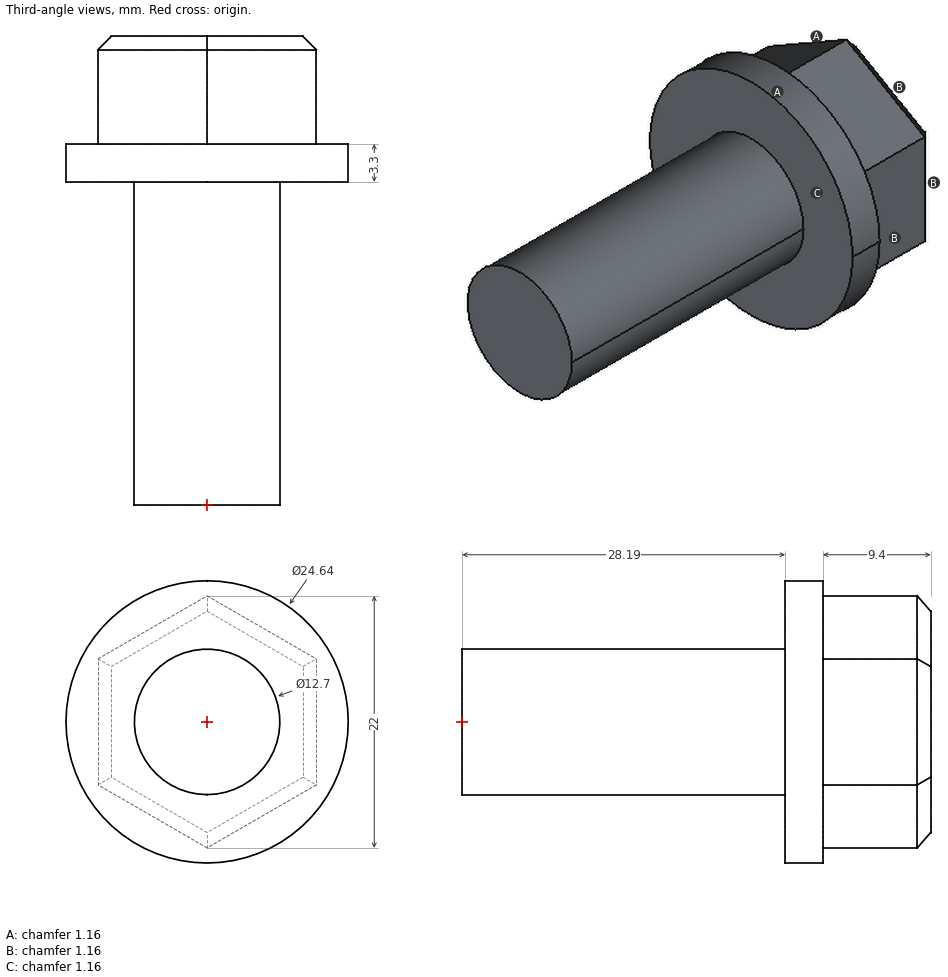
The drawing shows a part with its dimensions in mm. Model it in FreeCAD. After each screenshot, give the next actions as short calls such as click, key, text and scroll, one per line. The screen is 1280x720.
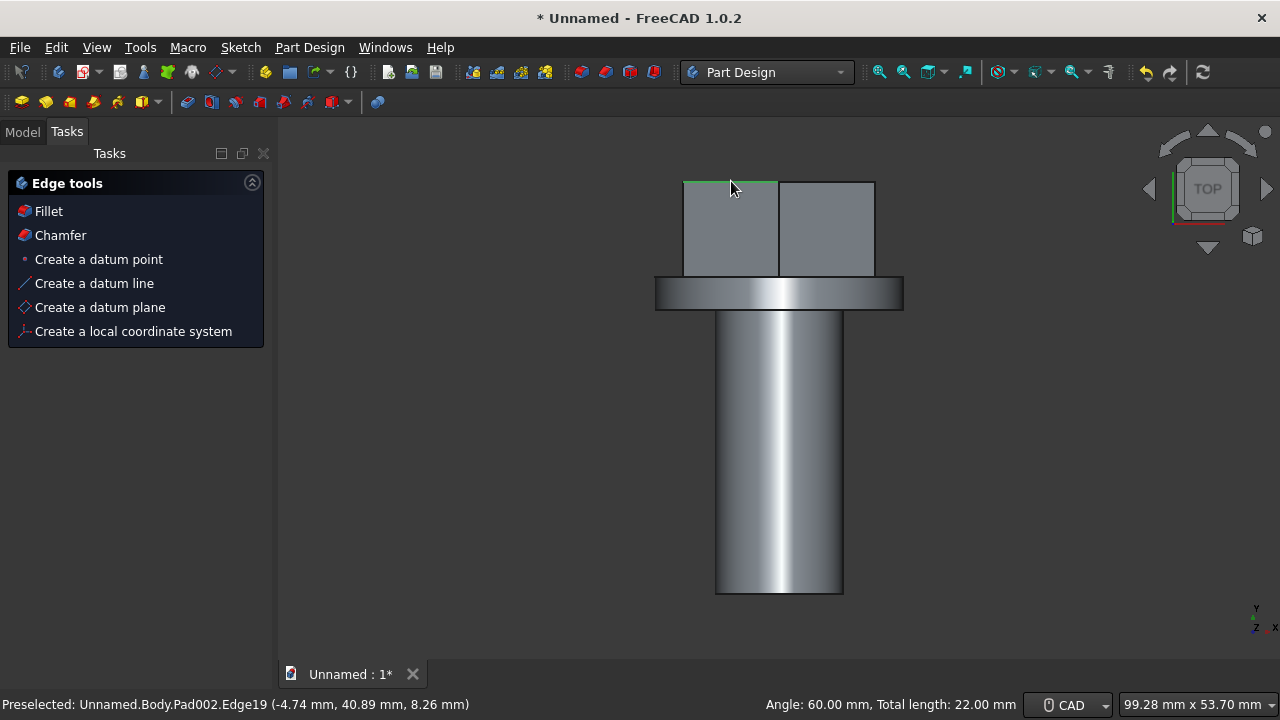
click(606, 72)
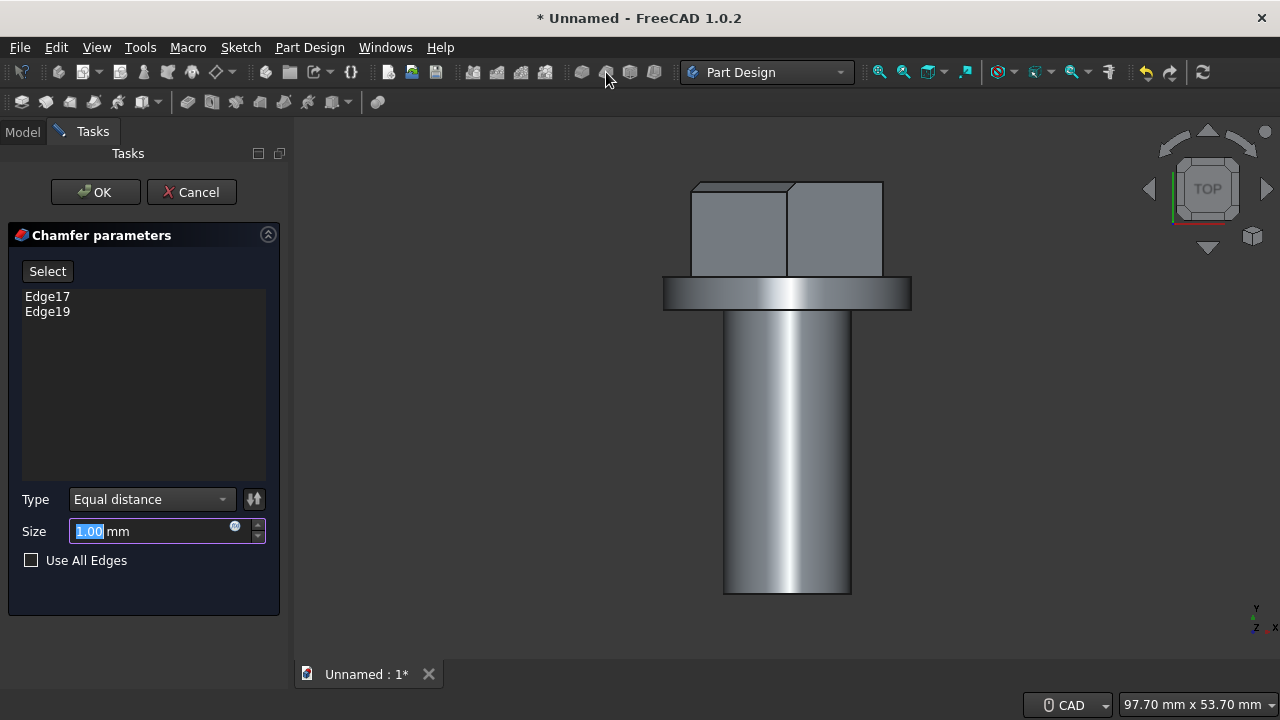
text(1.16)
key(Tab)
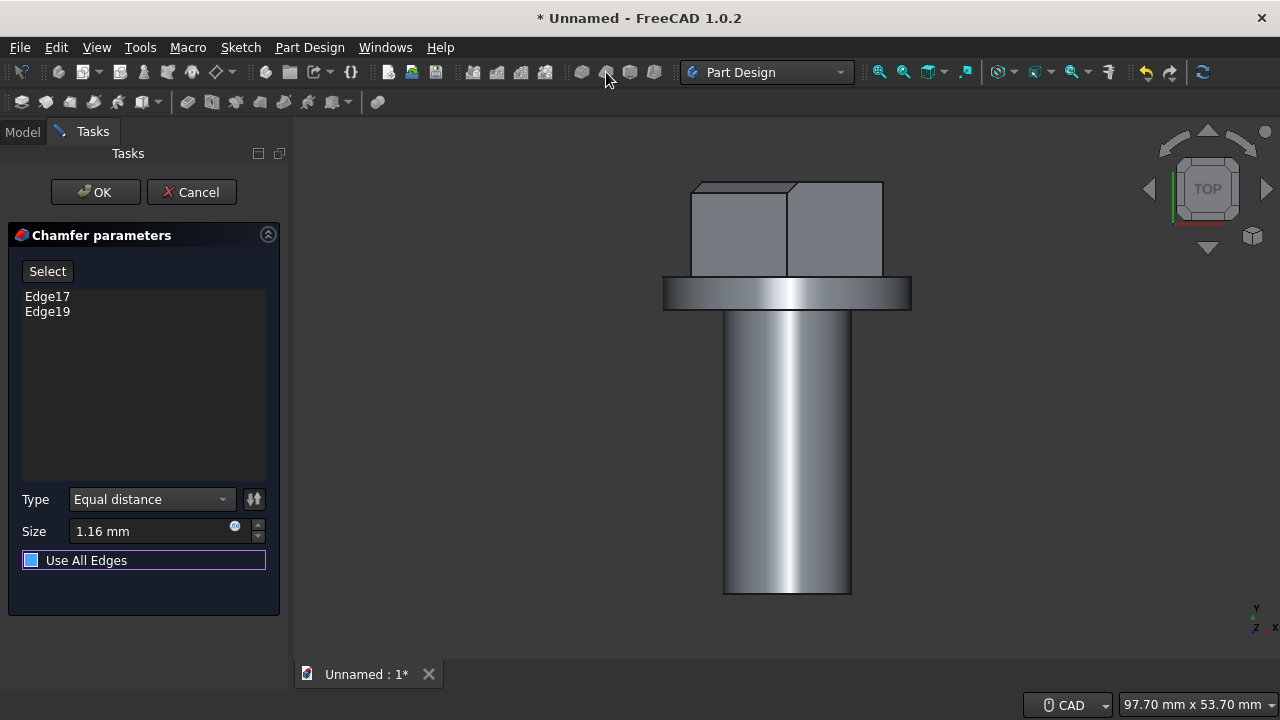
click(96, 192)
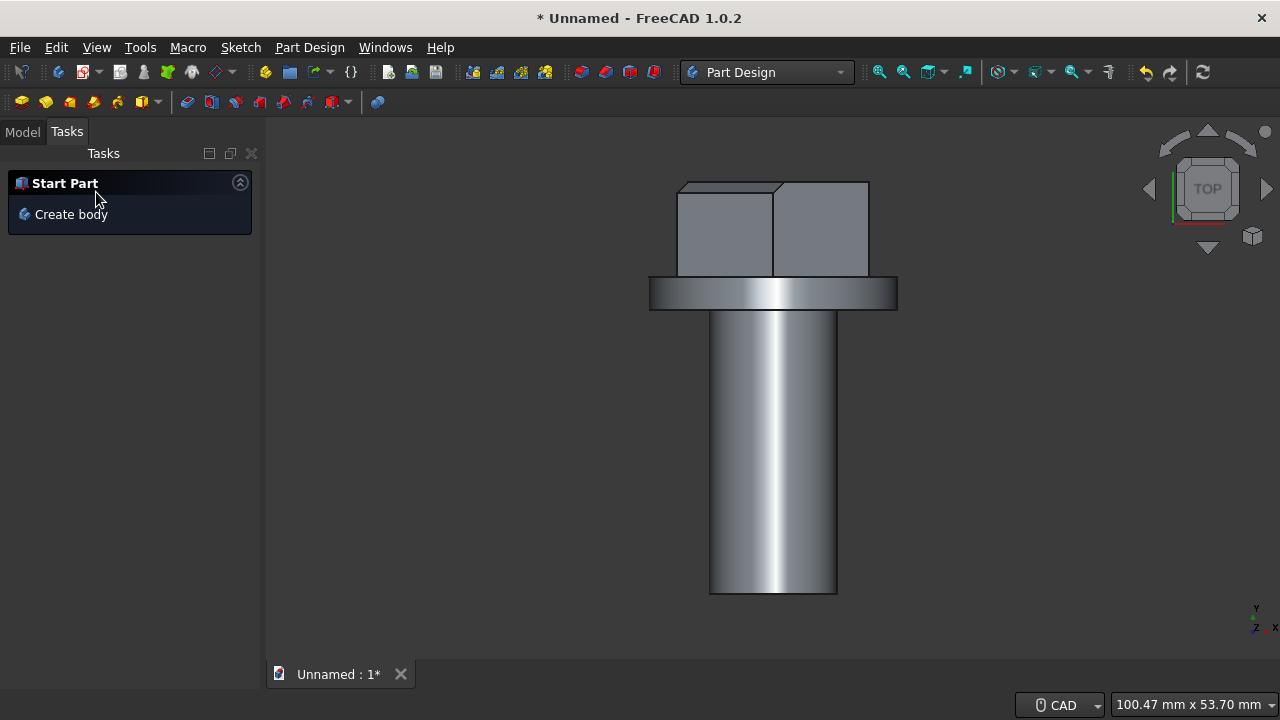
click(827, 181)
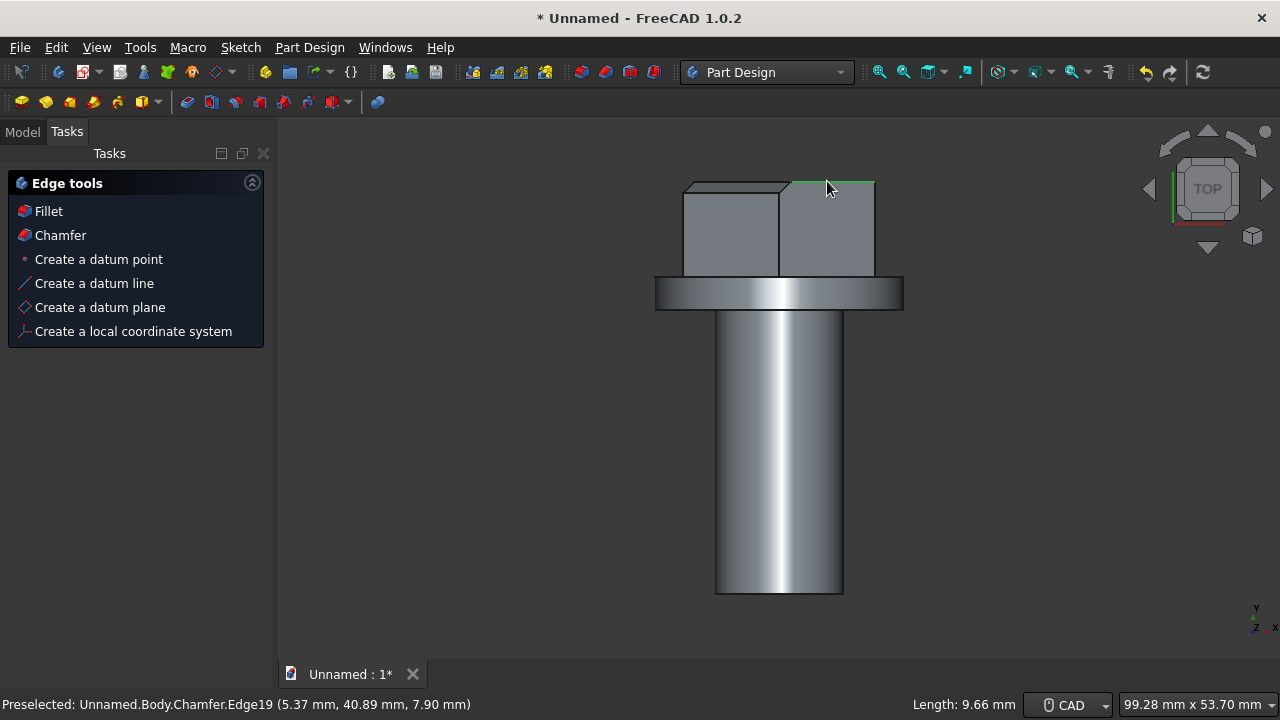
key(0)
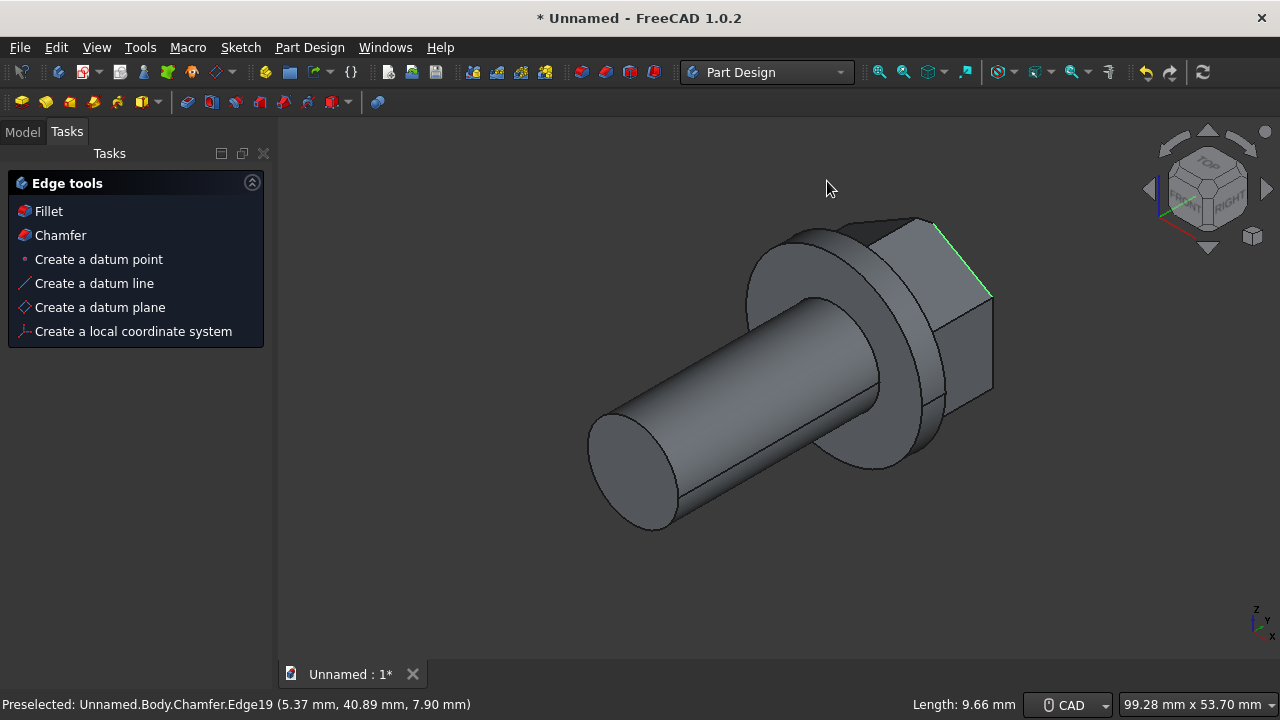
key(2)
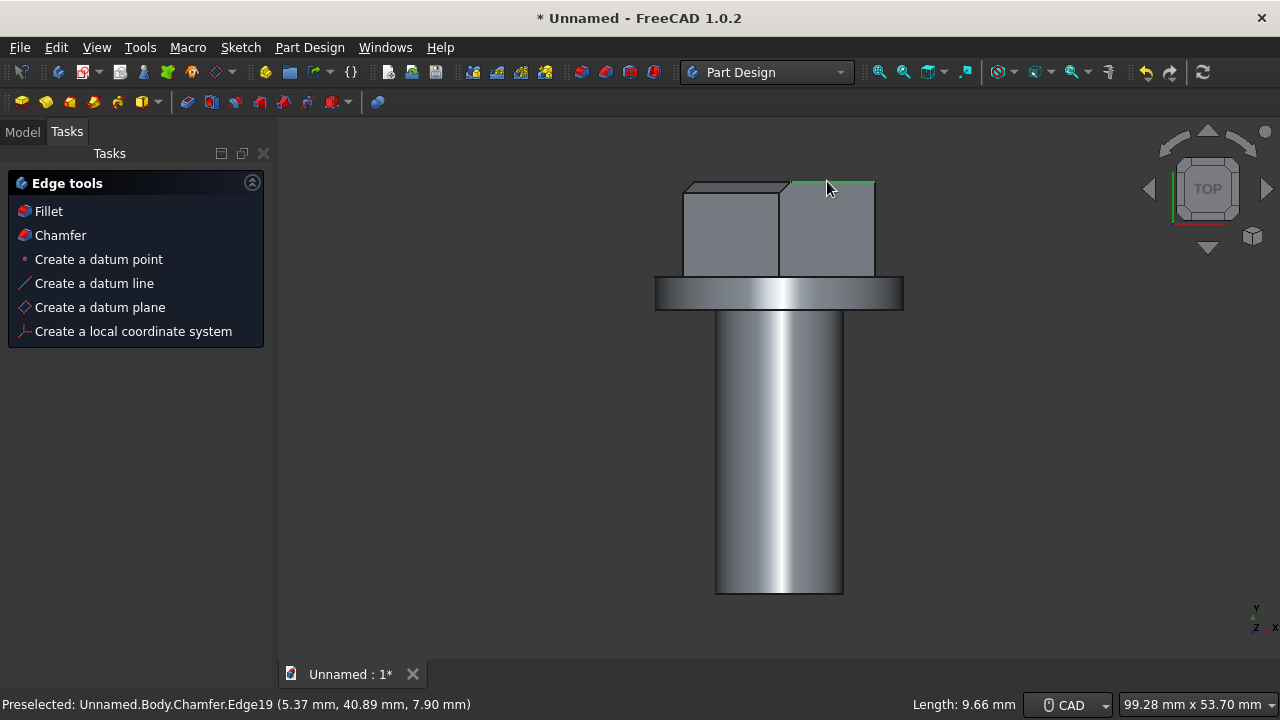
key(1)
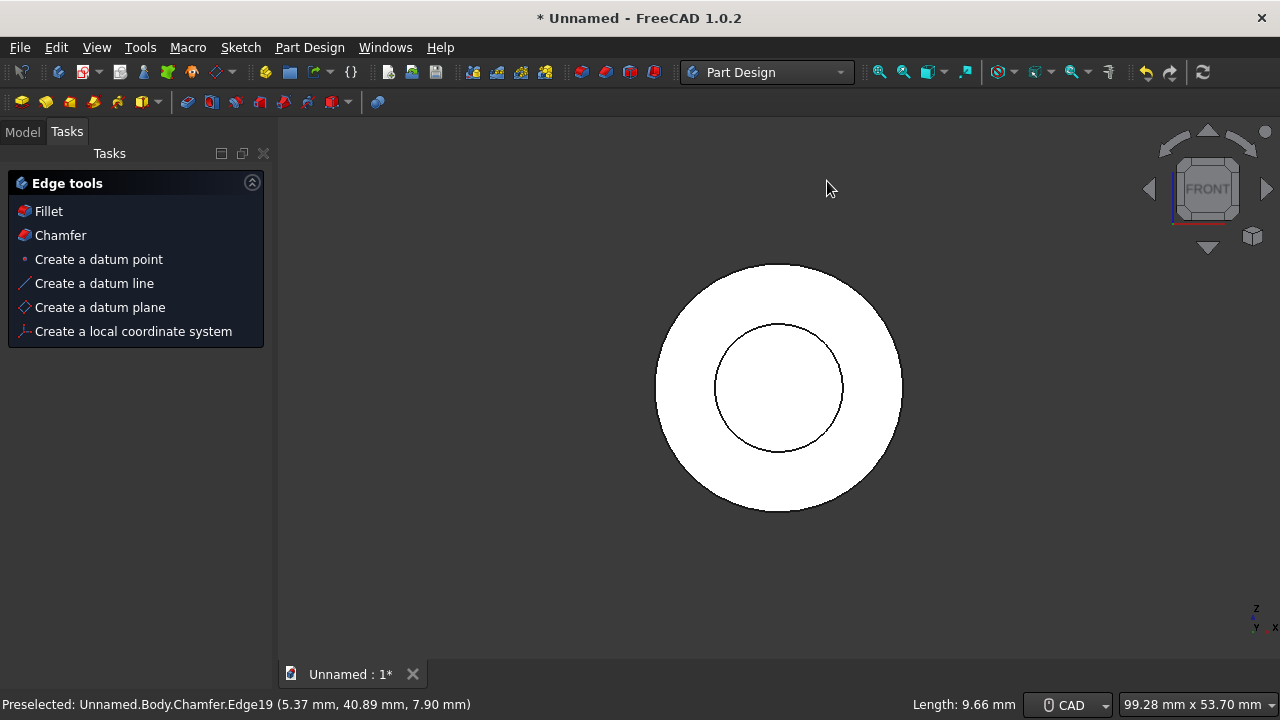
key(3)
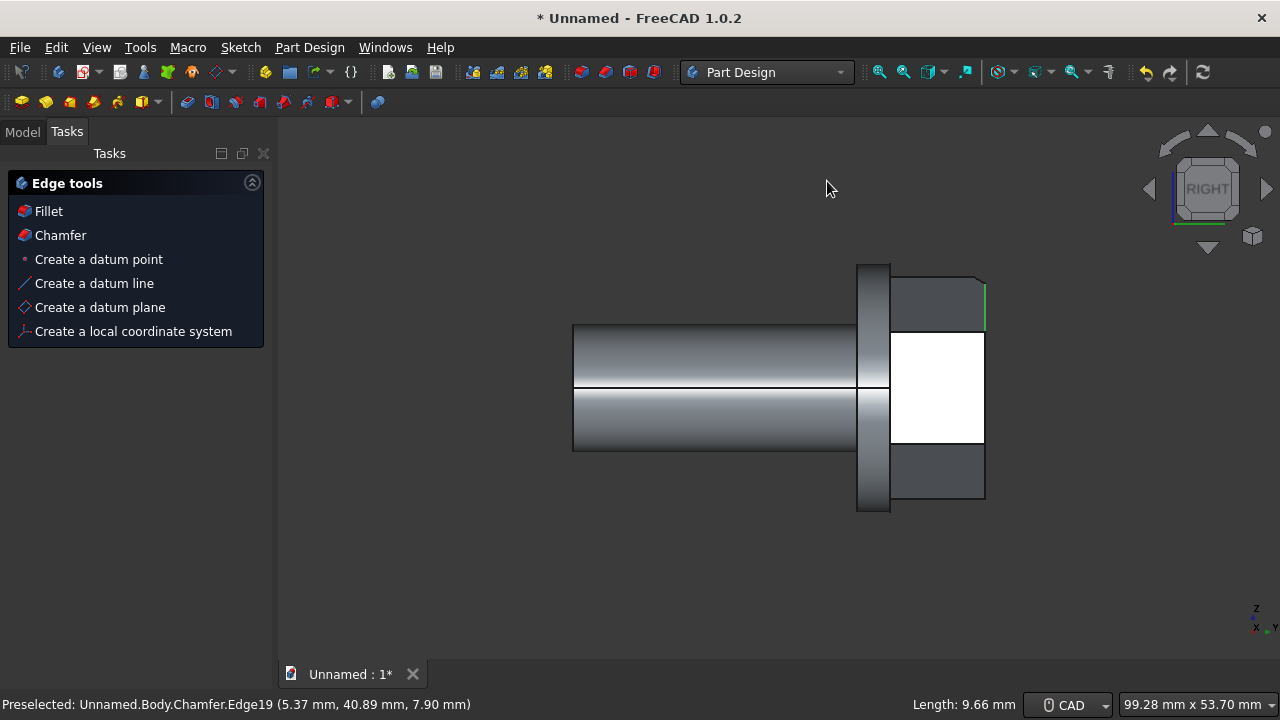
click(985, 470, ctrl)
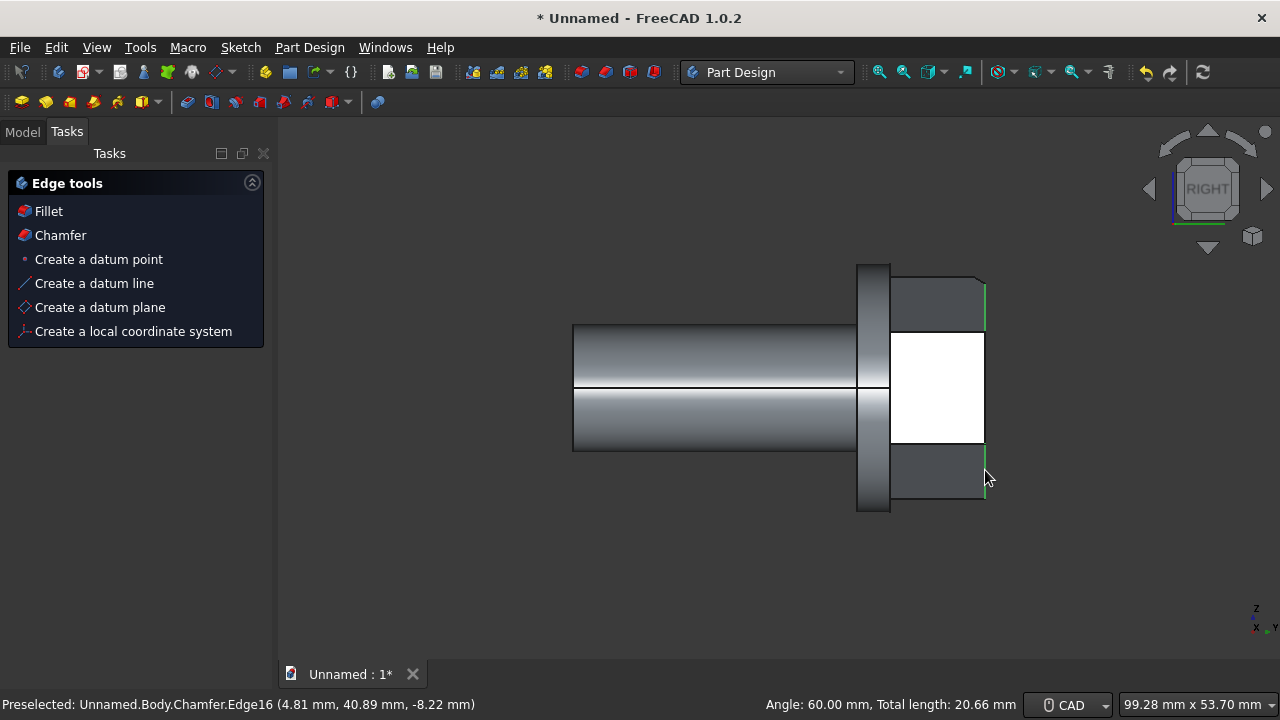
click(985, 387, ctrl)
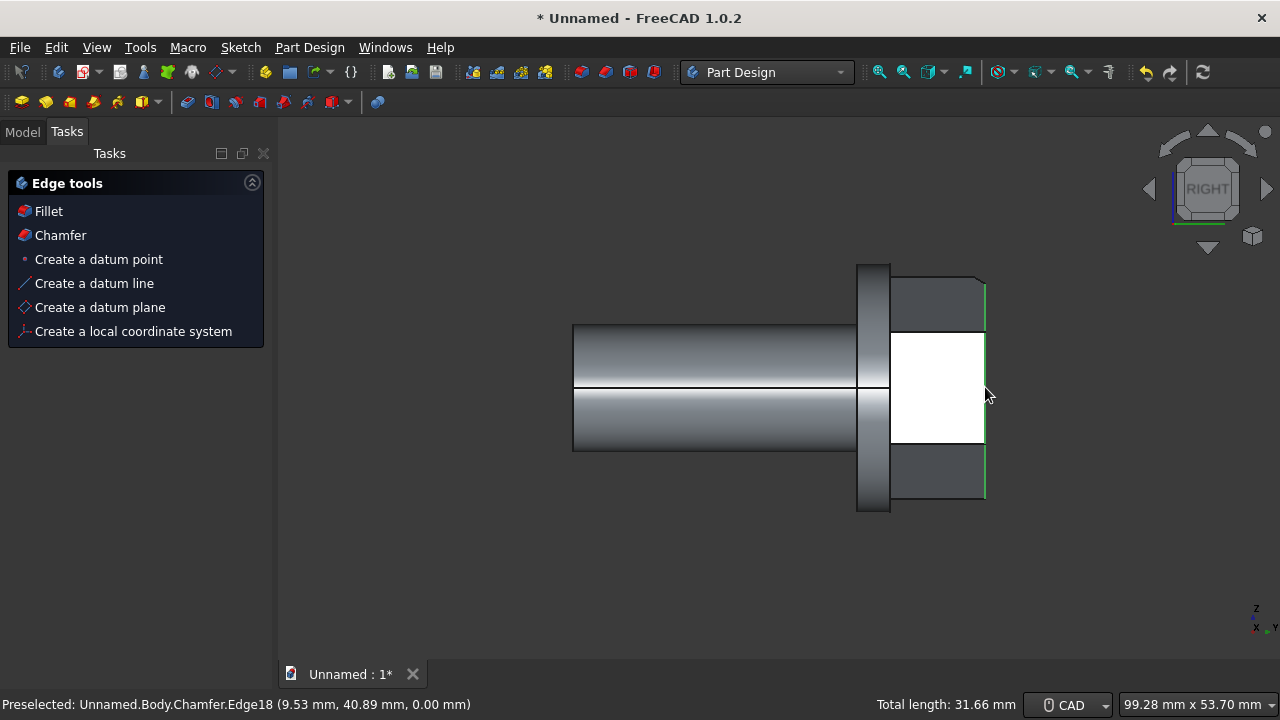
click(606, 72)